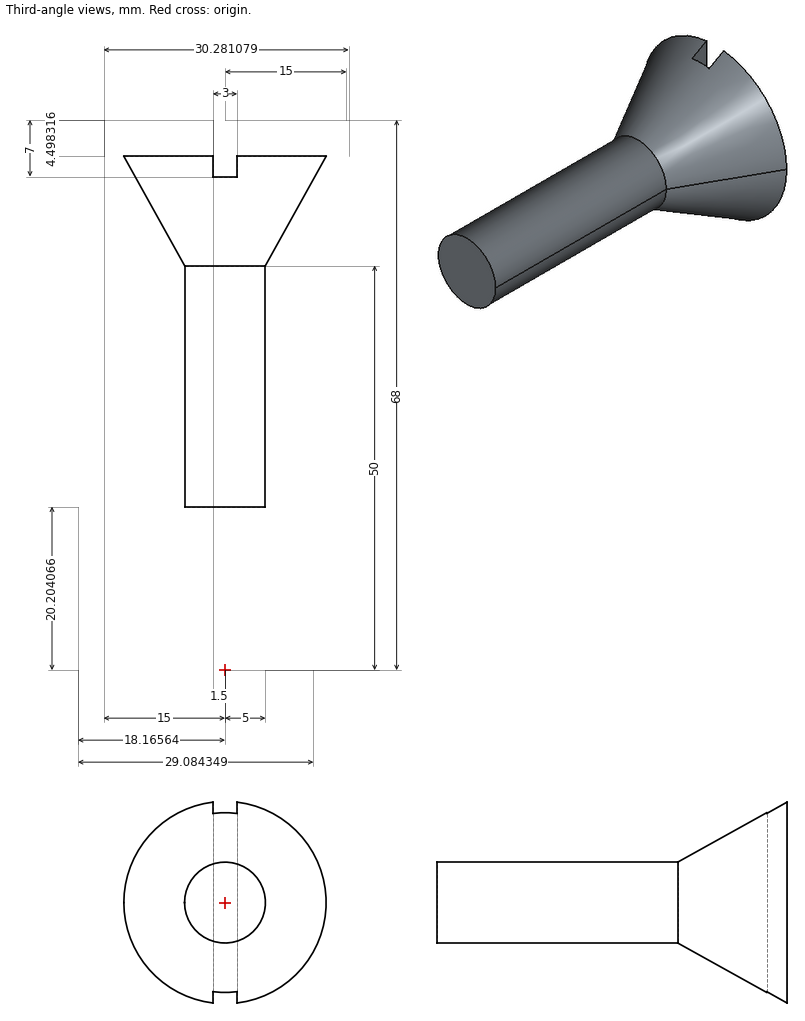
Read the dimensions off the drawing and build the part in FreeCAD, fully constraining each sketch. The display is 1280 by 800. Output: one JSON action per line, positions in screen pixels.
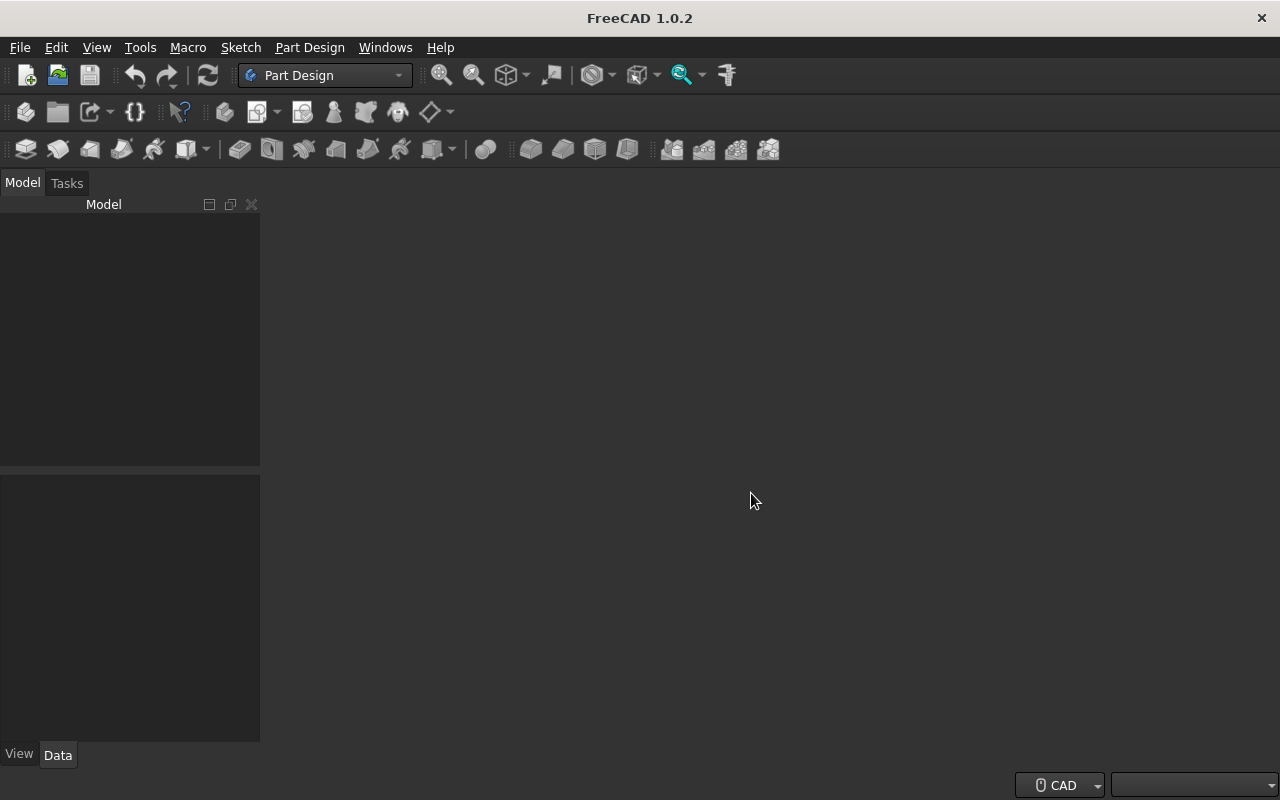
{"action": "key", "text": "ctrl+n"}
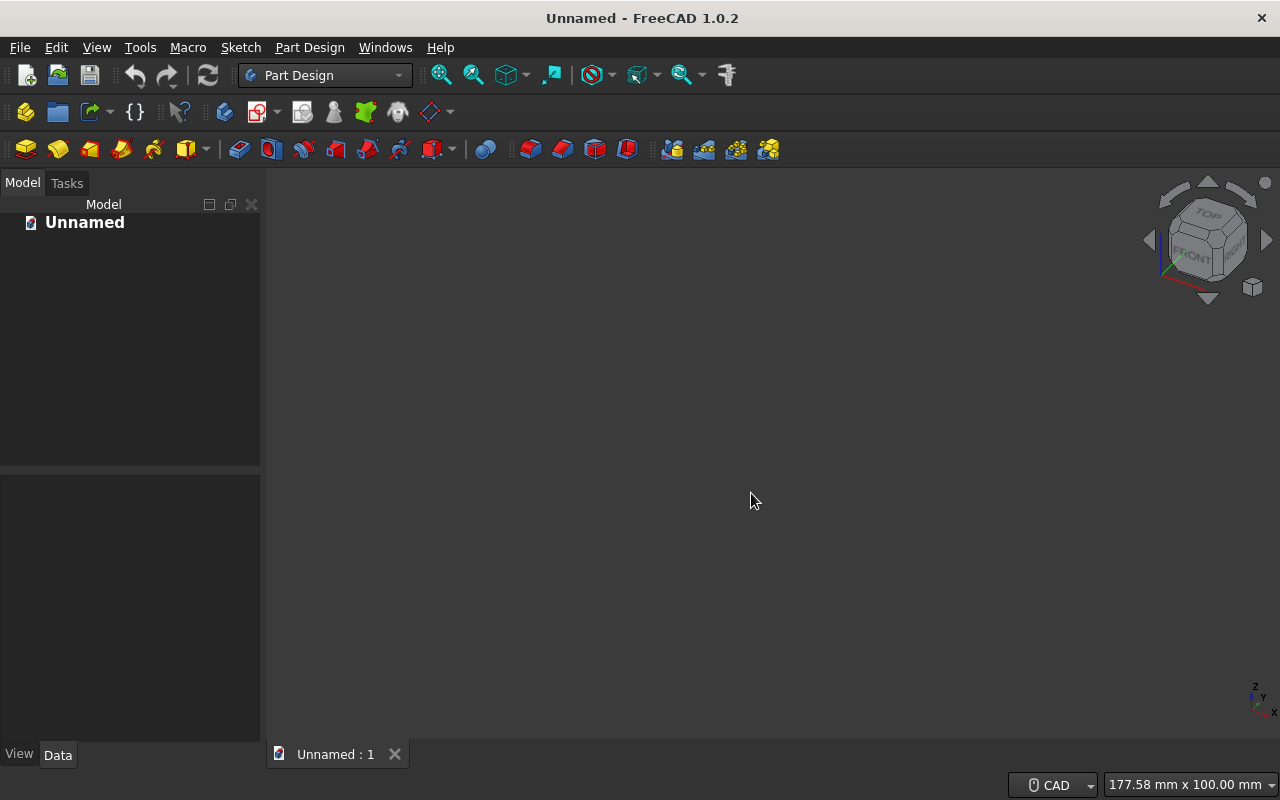
{"action": "left_click", "coordinate": [258, 112]}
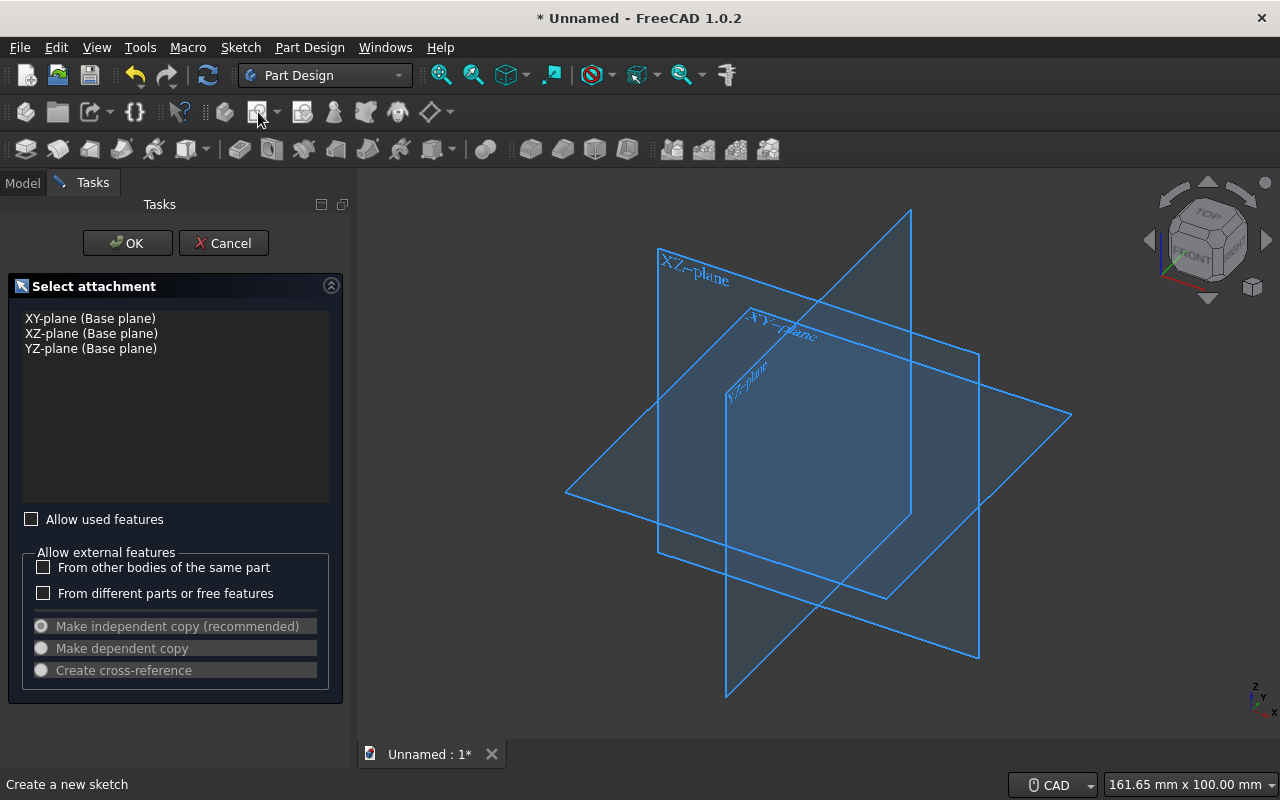
{"action": "left_click", "coordinate": [82, 318]}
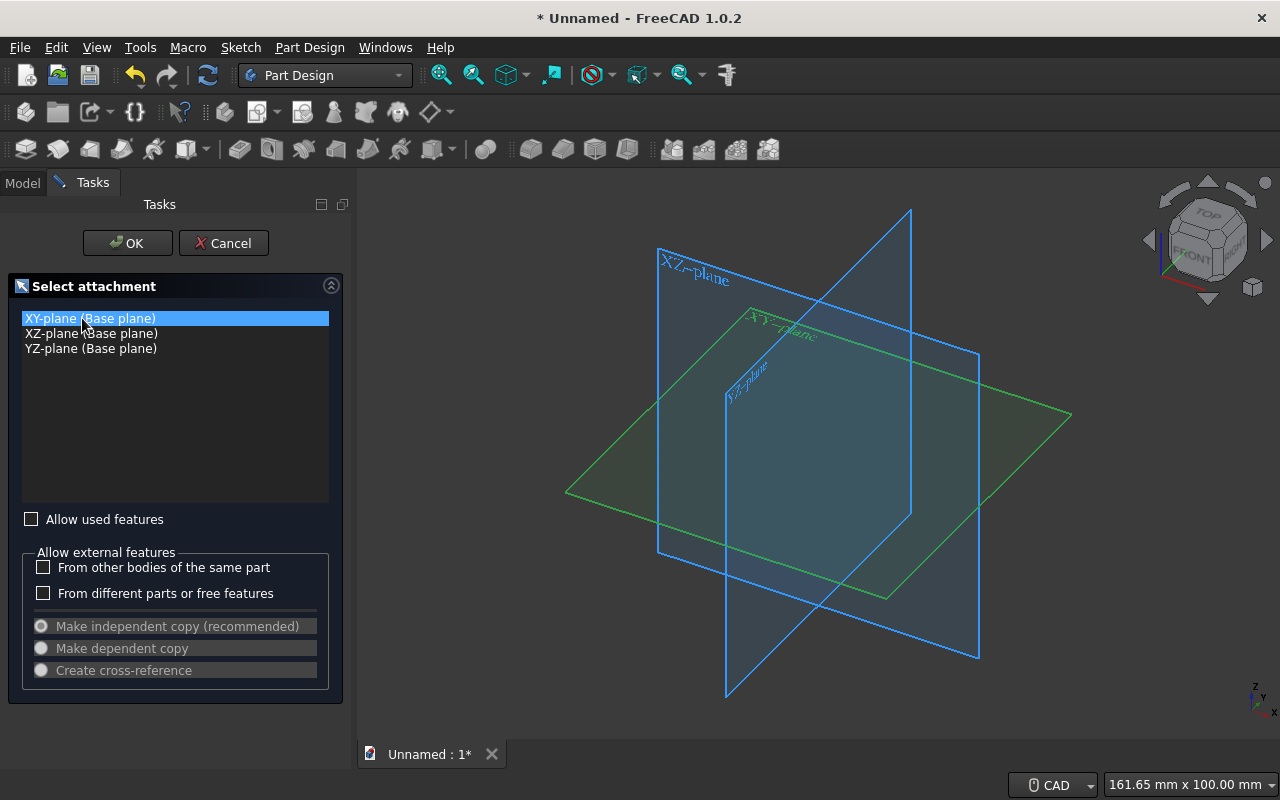
{"action": "left_click", "coordinate": [128, 243]}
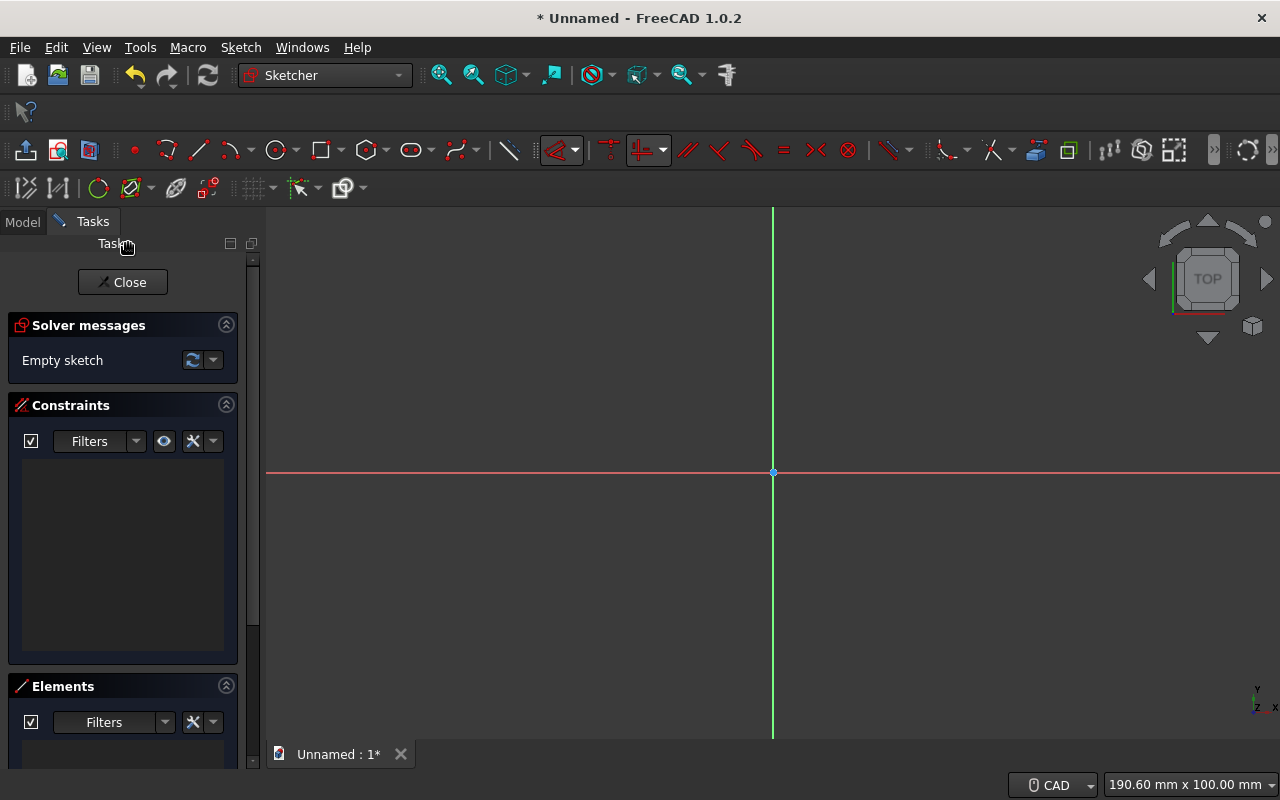
{"action": "scroll", "coordinate": [484, 711], "scroll_direction": "down", "scroll_amount": 2}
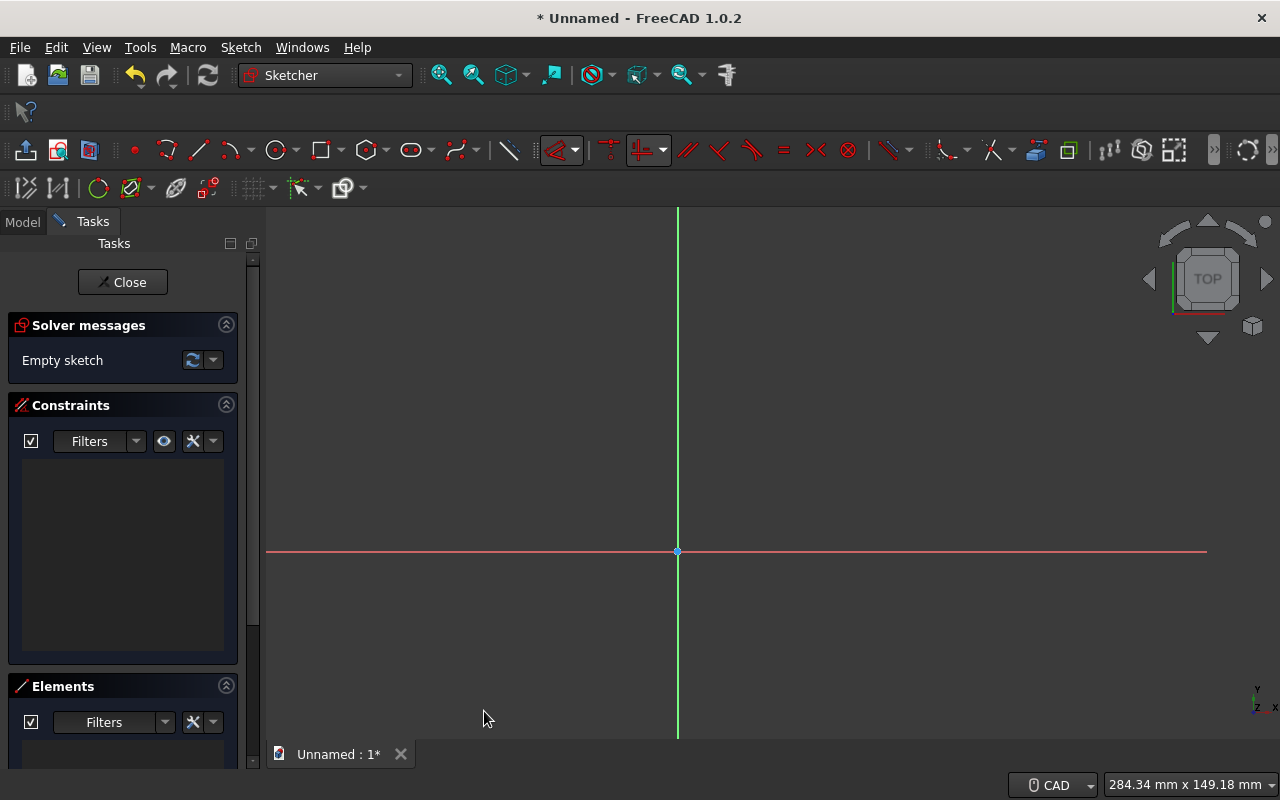
{"action": "scroll", "coordinate": [705, 344], "scroll_direction": "up", "scroll_amount": 2}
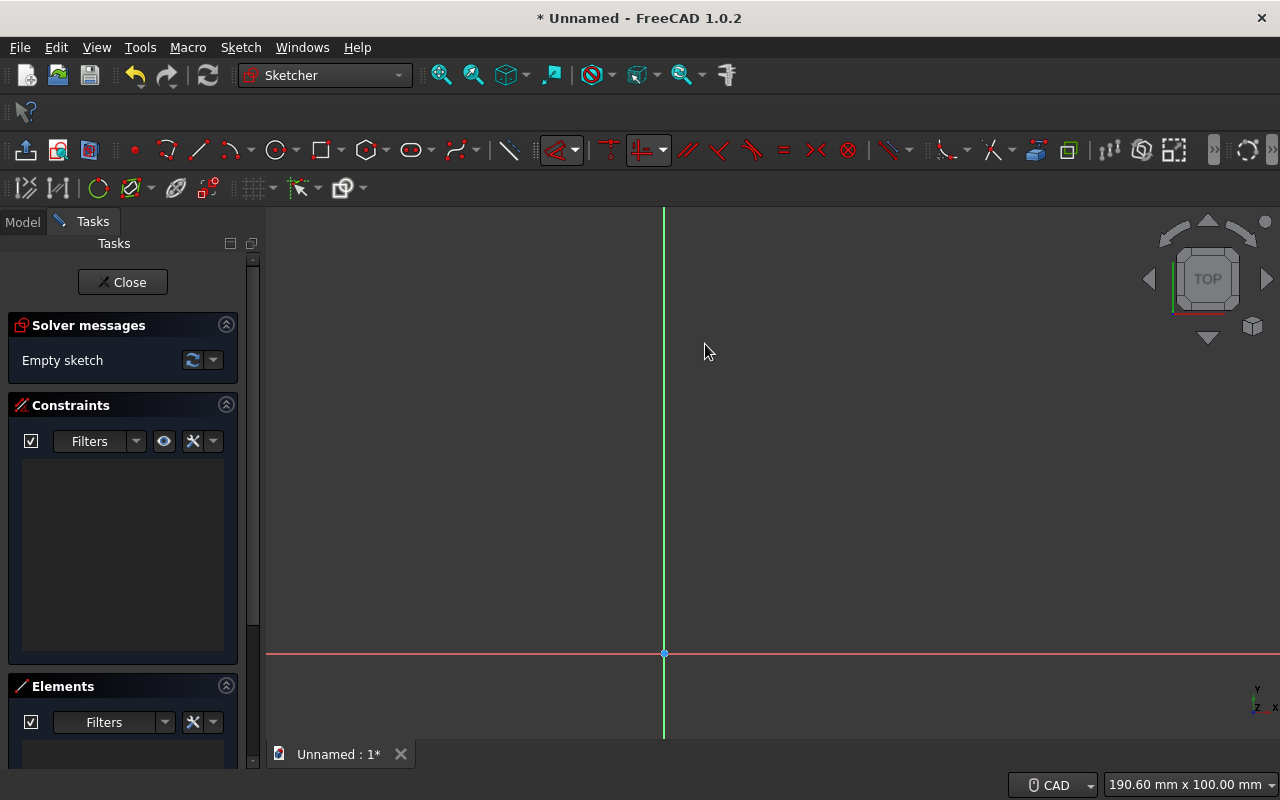
{"action": "left_click", "coordinate": [168, 150]}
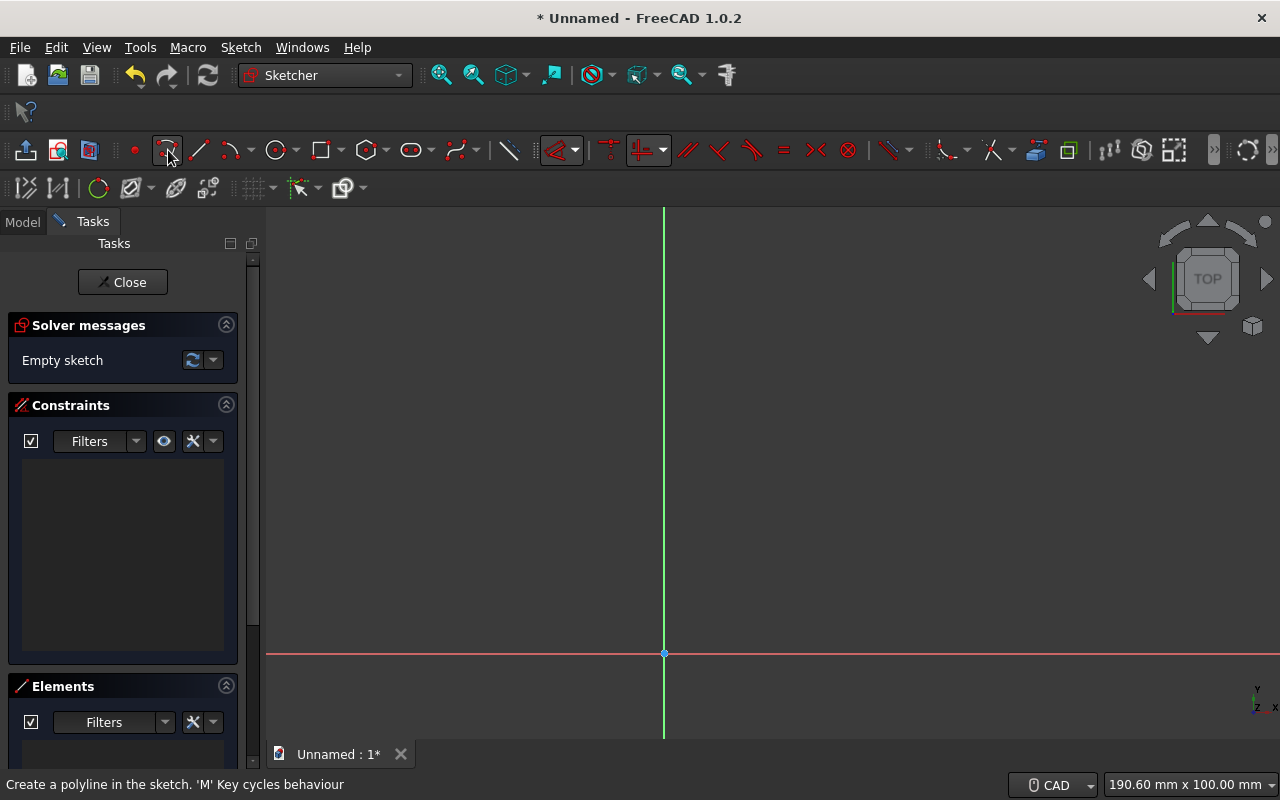
{"action": "left_click", "coordinate": [664, 654]}
{"action": "left_click", "coordinate": [691, 645]}
{"action": "left_click", "coordinate": [691, 388]}
{"action": "left_click", "coordinate": [744, 292]}
{"action": "left_click", "coordinate": [673, 292]}
{"action": "left_click", "coordinate": [664, 654]}
{"action": "key", "text": "Escape"}
{"action": "key", "text": "Escape"}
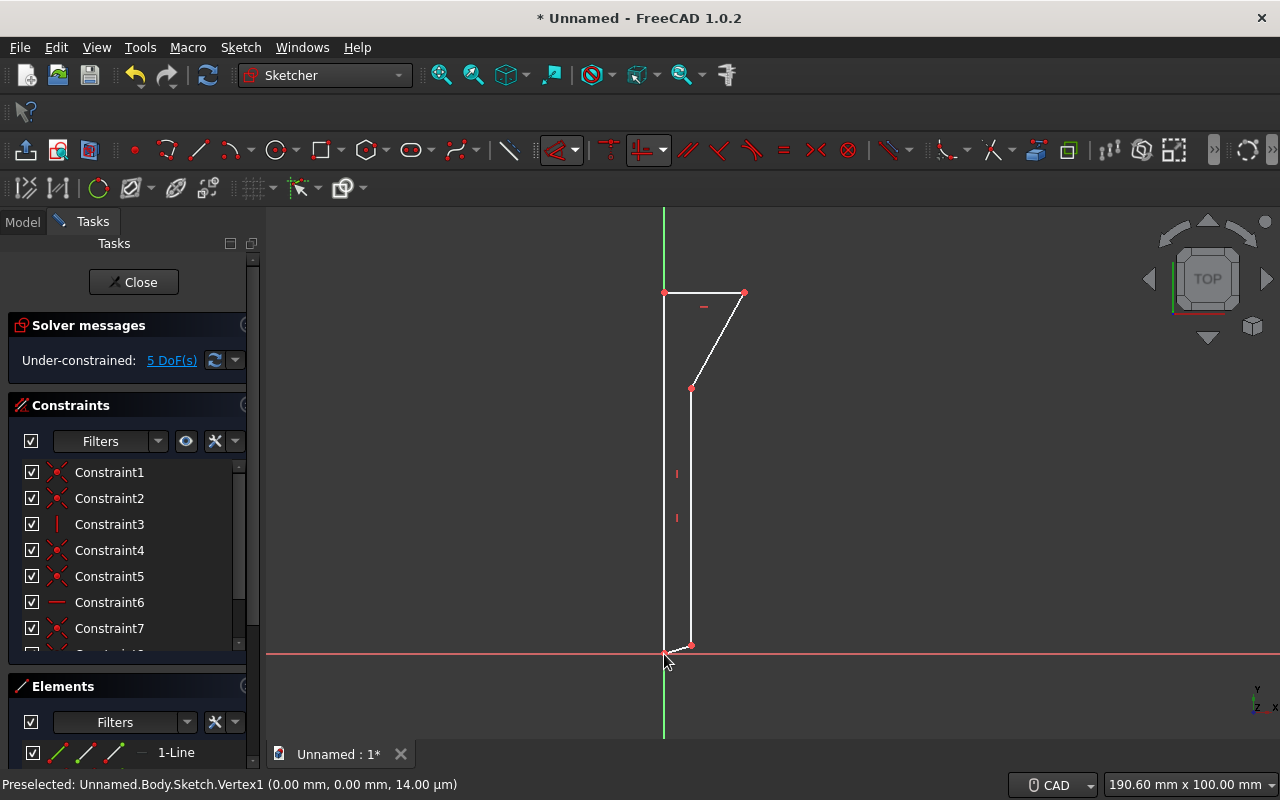
{"action": "scroll", "coordinate": [675, 651], "scroll_direction": "up", "scroll_amount": 2}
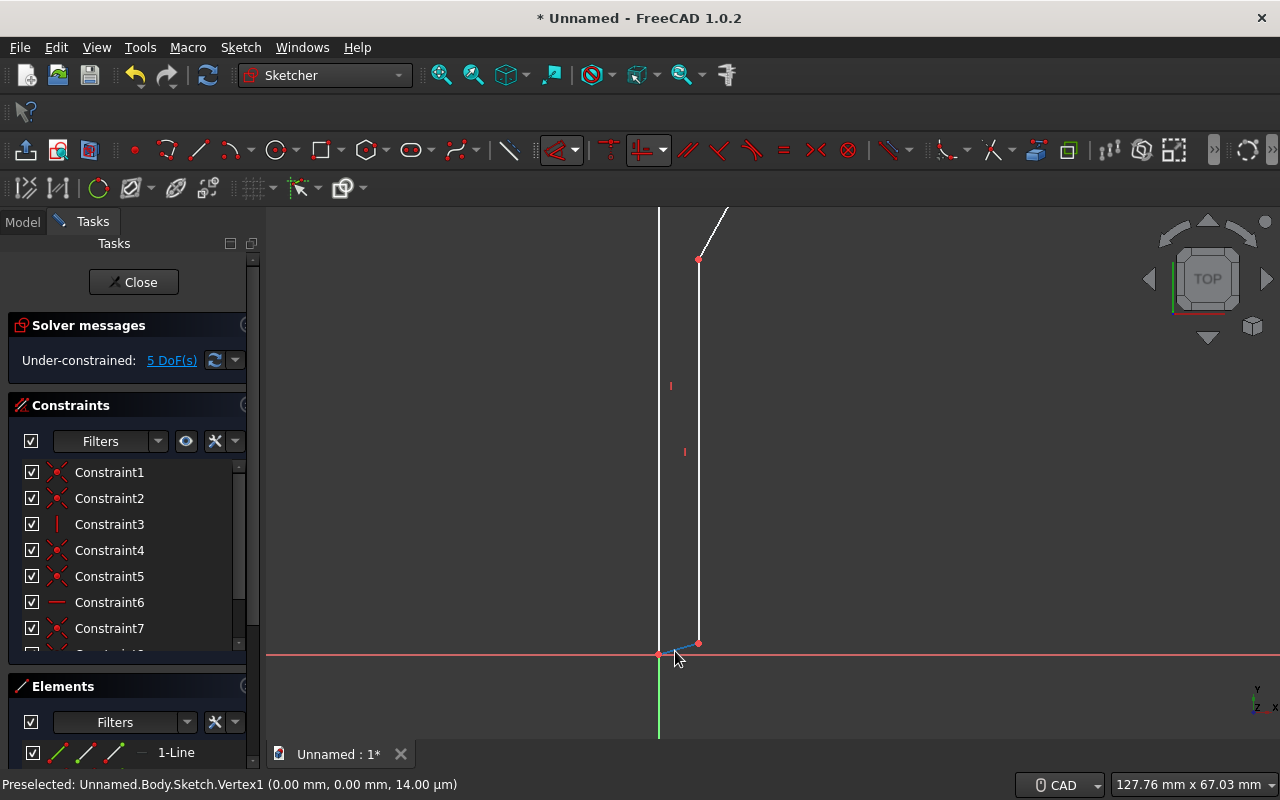
{"action": "left_click", "coordinate": [675, 650]}